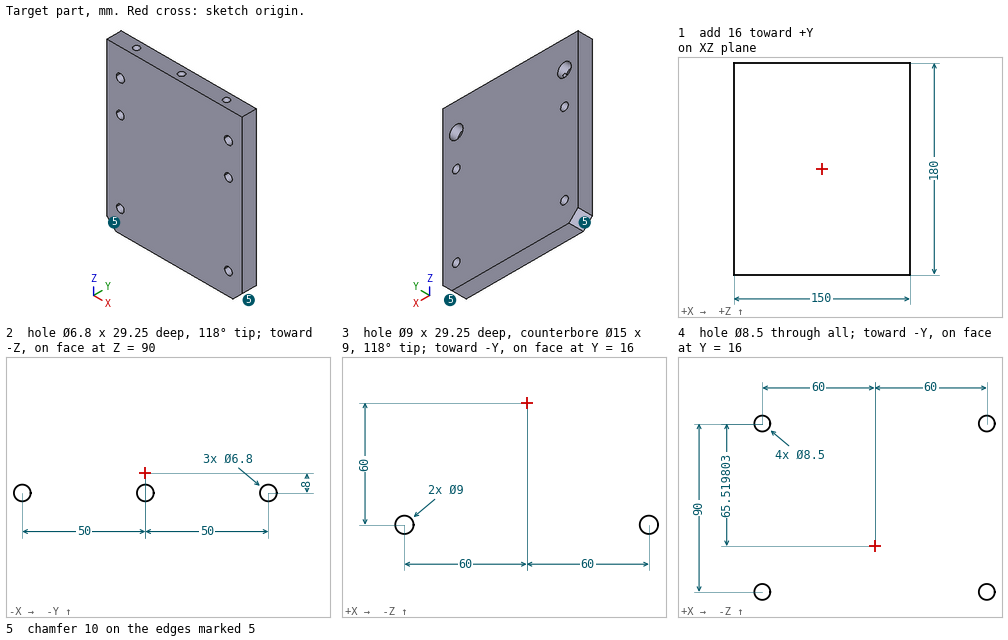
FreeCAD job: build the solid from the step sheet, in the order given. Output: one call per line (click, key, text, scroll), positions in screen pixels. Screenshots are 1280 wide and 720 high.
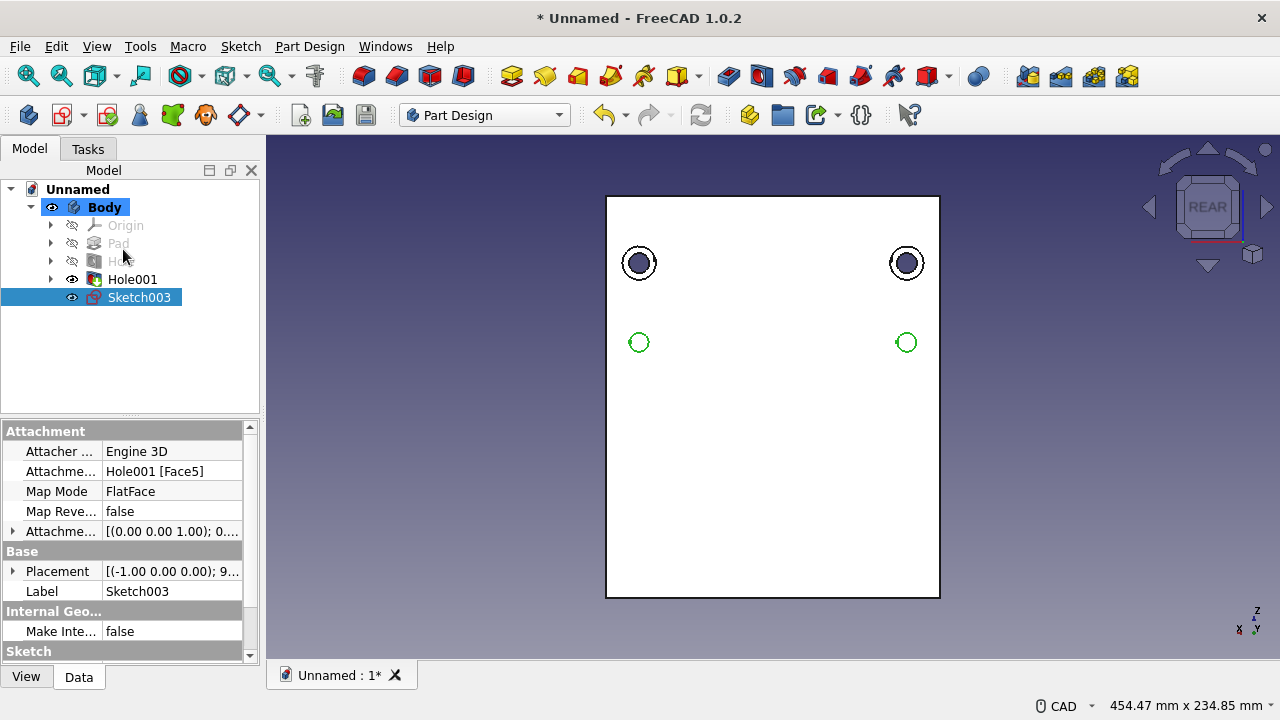
click(762, 76)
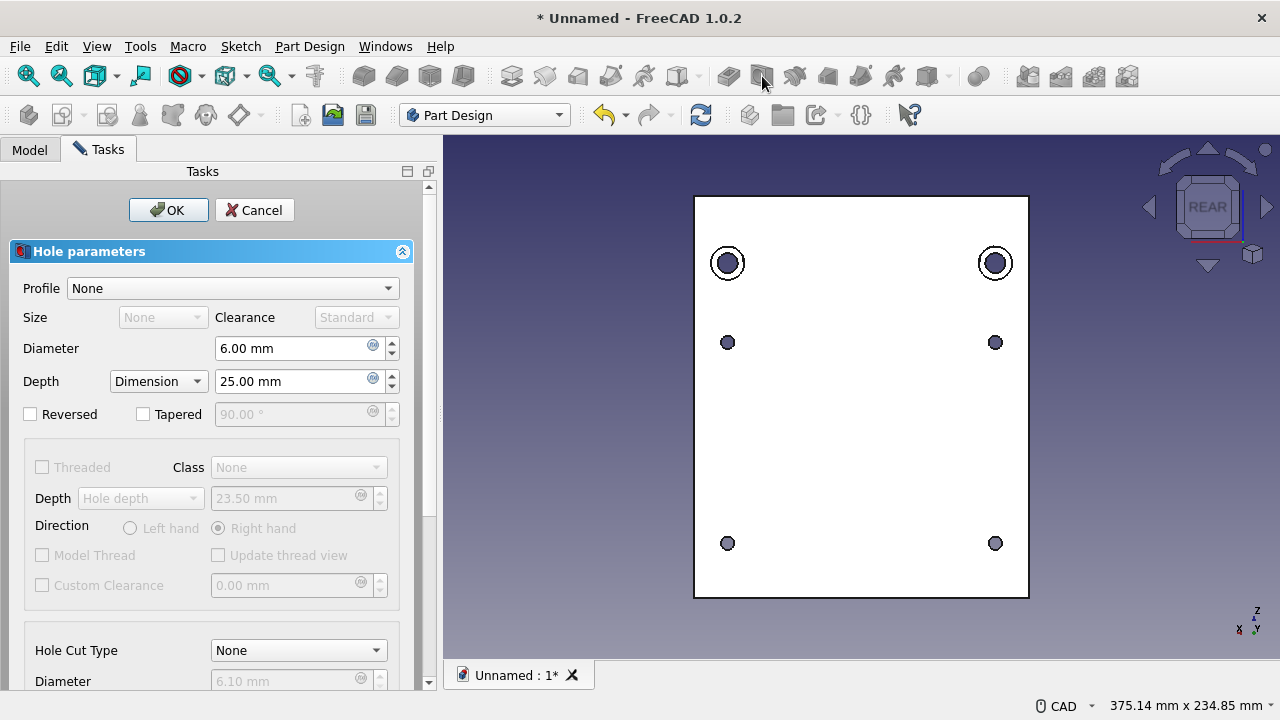
triple_click(300, 348)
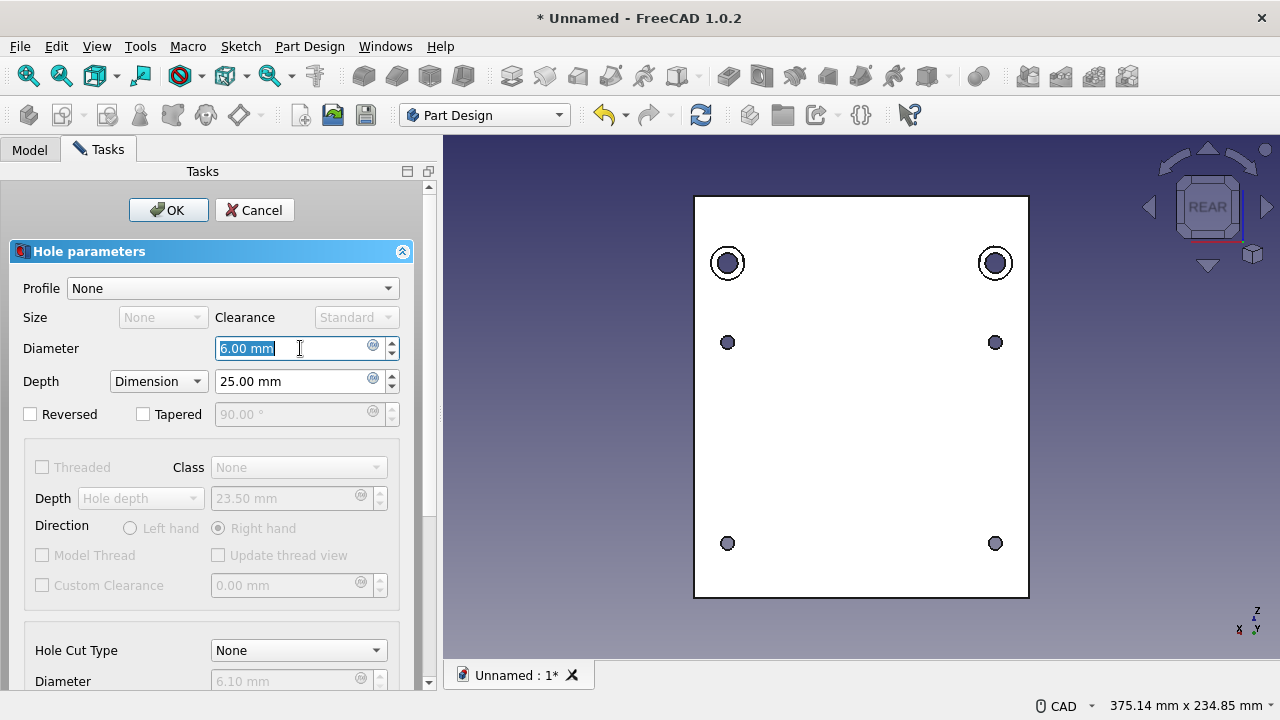
text(8.5)
key(Tab)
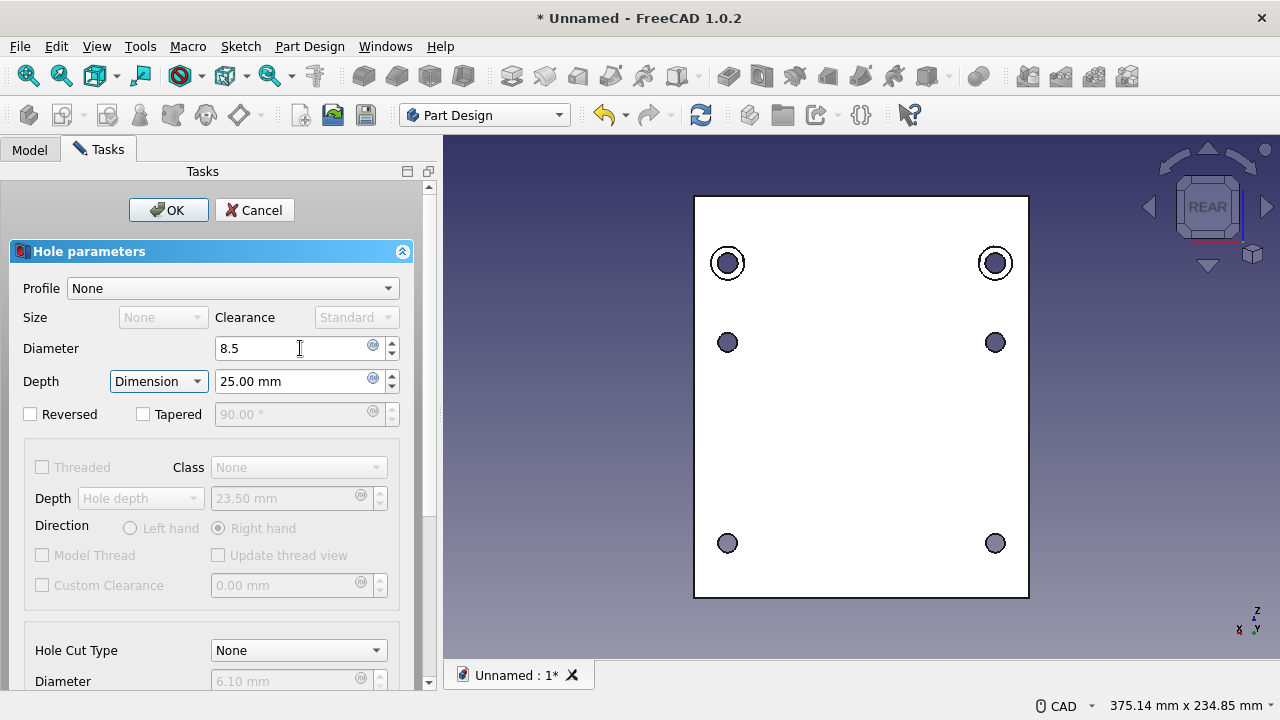
click(160, 382)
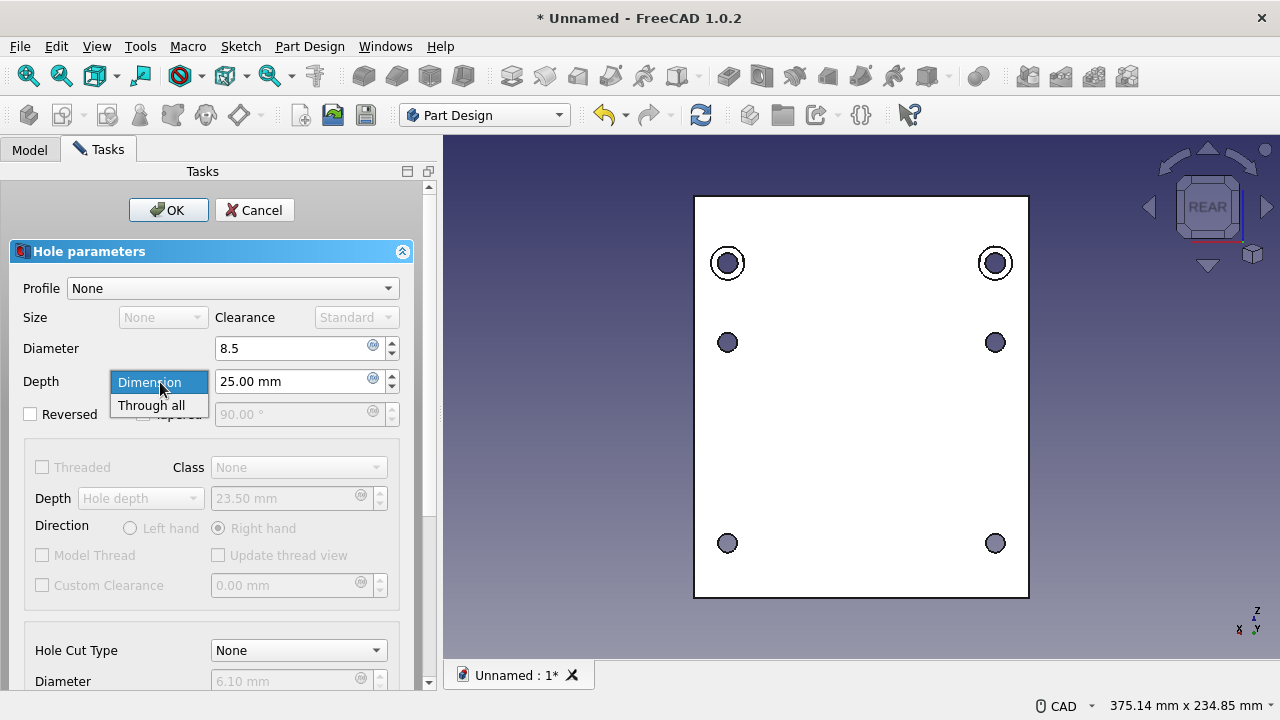
click(158, 406)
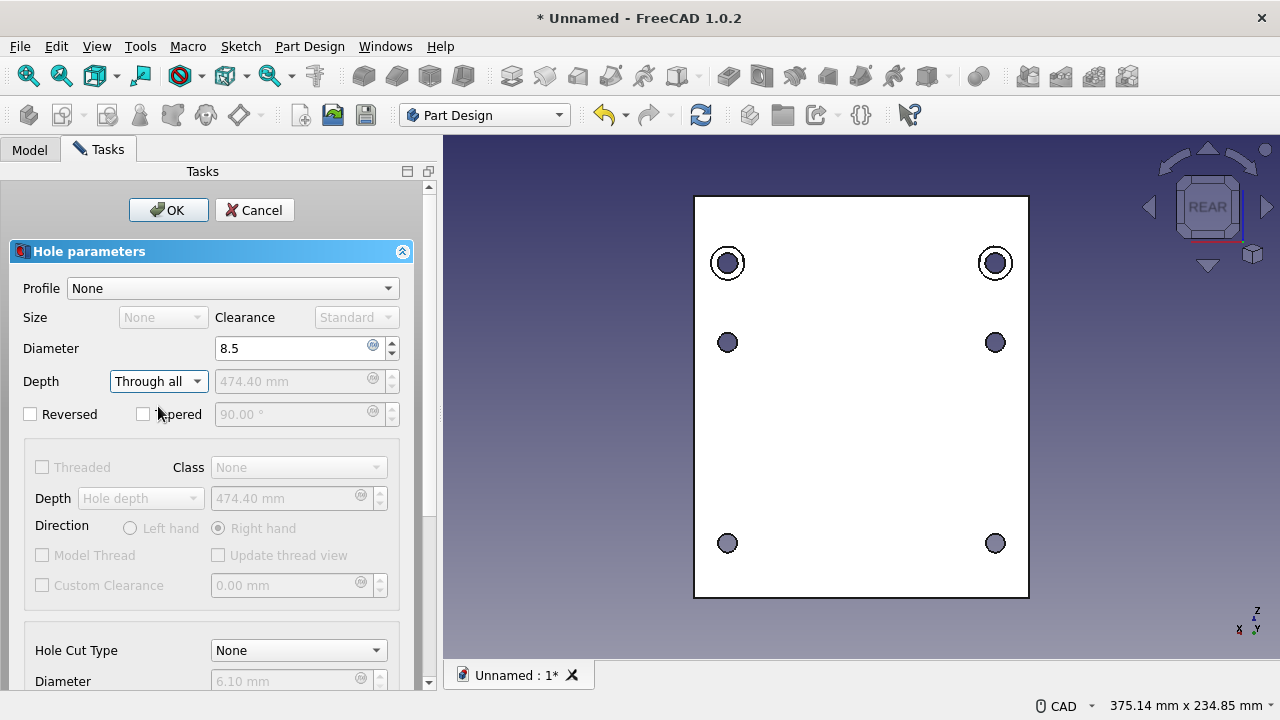
click(169, 210)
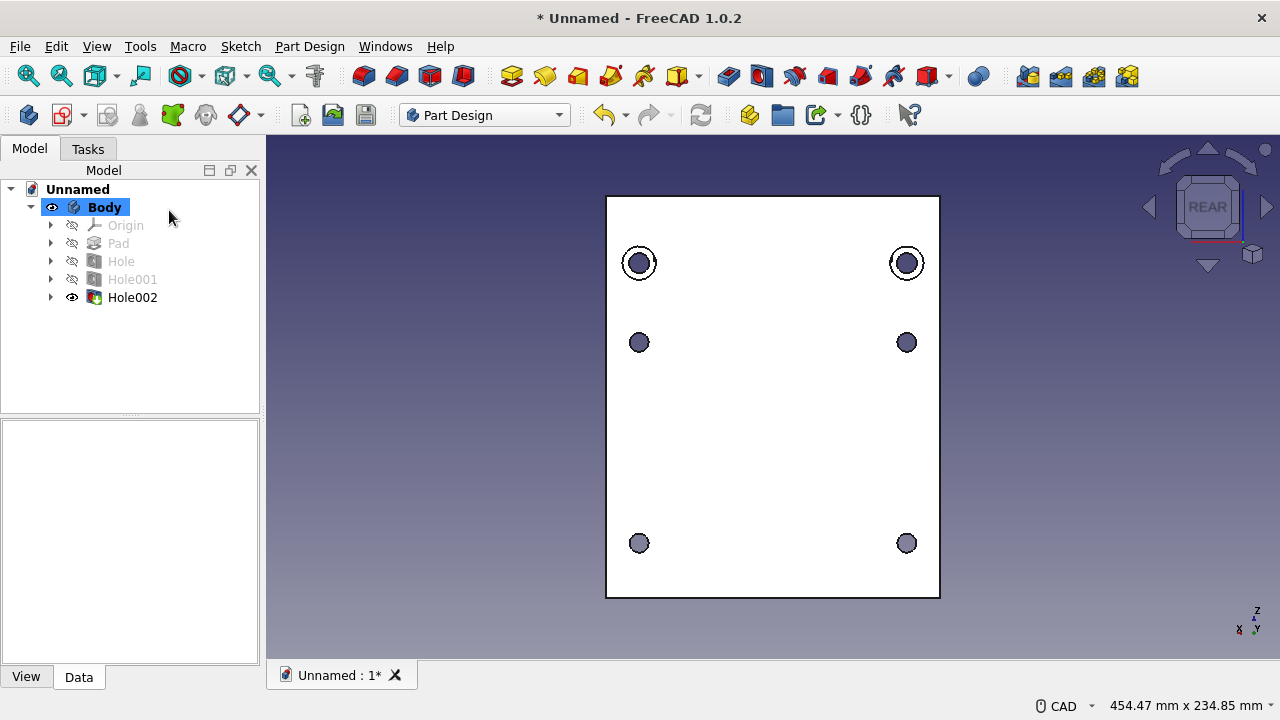
key(0)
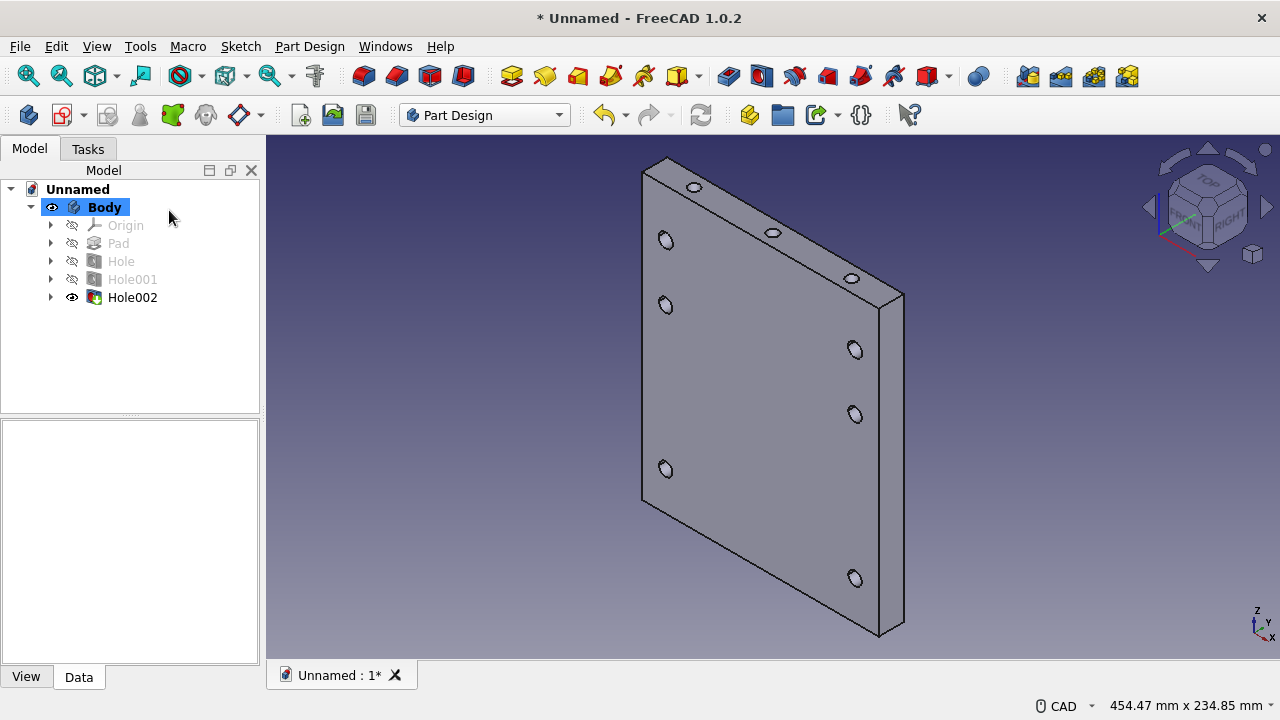
key(2)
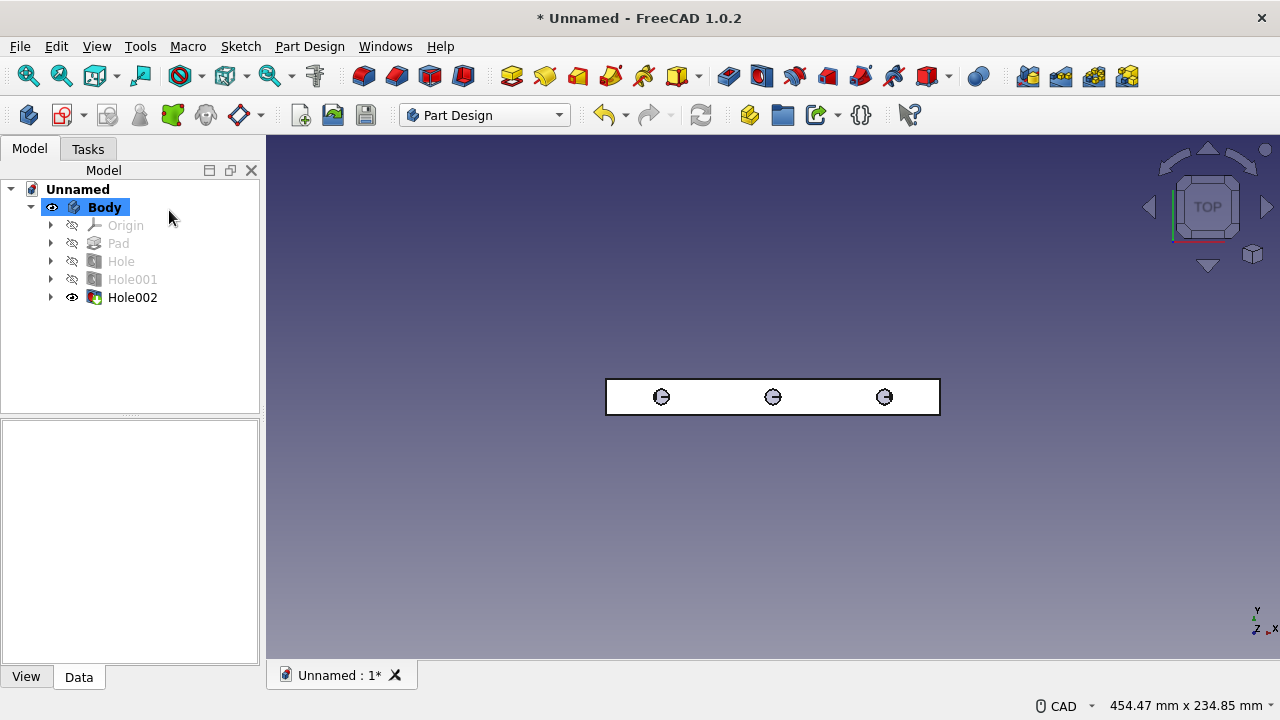
click(29, 76)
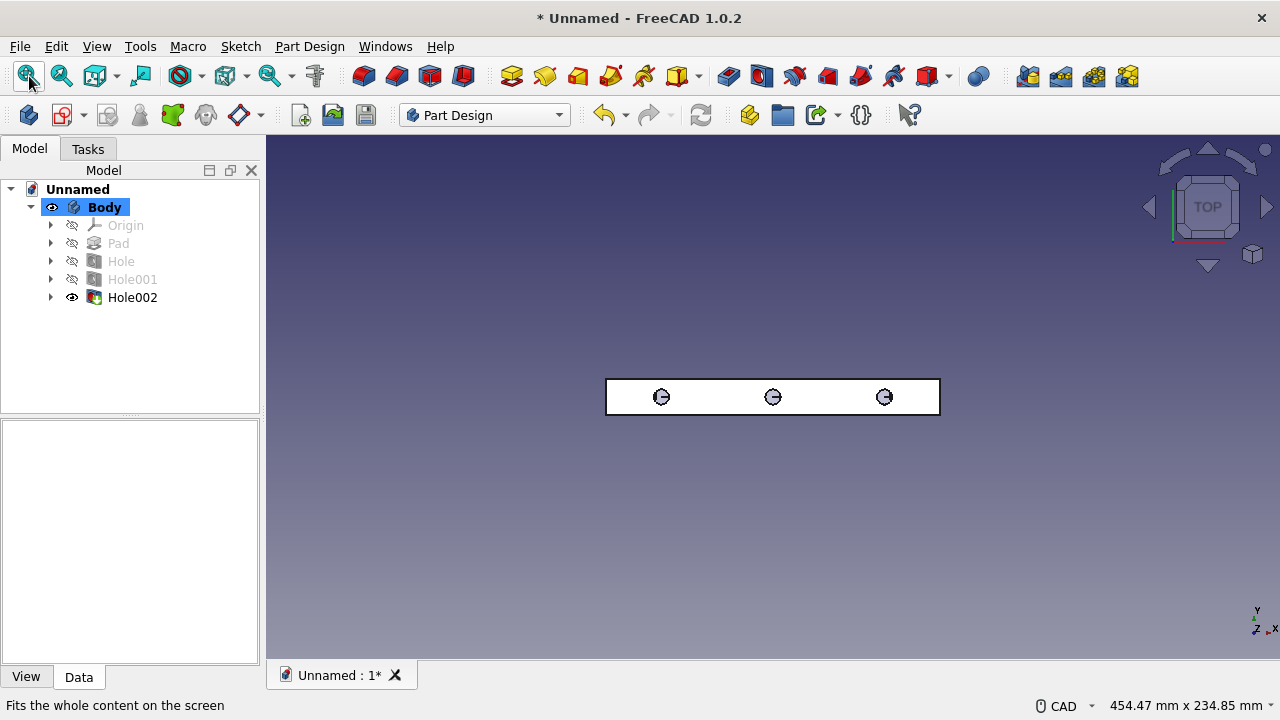
key(1)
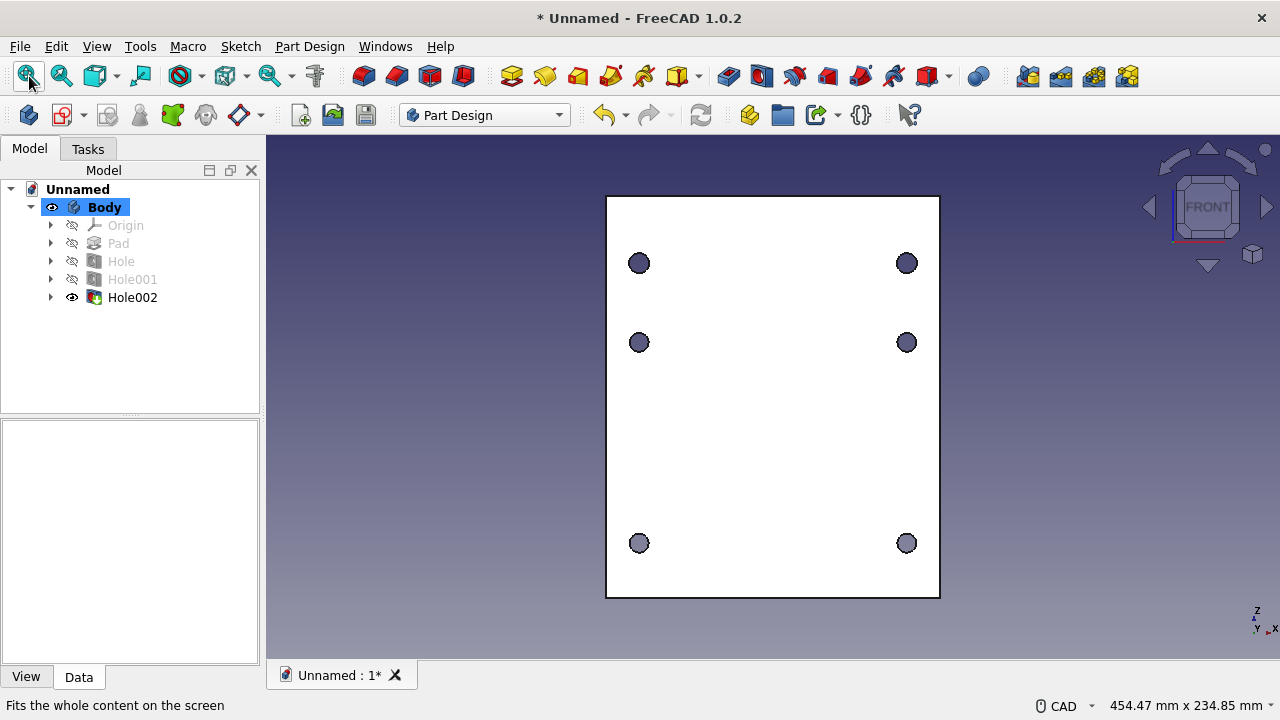
key(3)